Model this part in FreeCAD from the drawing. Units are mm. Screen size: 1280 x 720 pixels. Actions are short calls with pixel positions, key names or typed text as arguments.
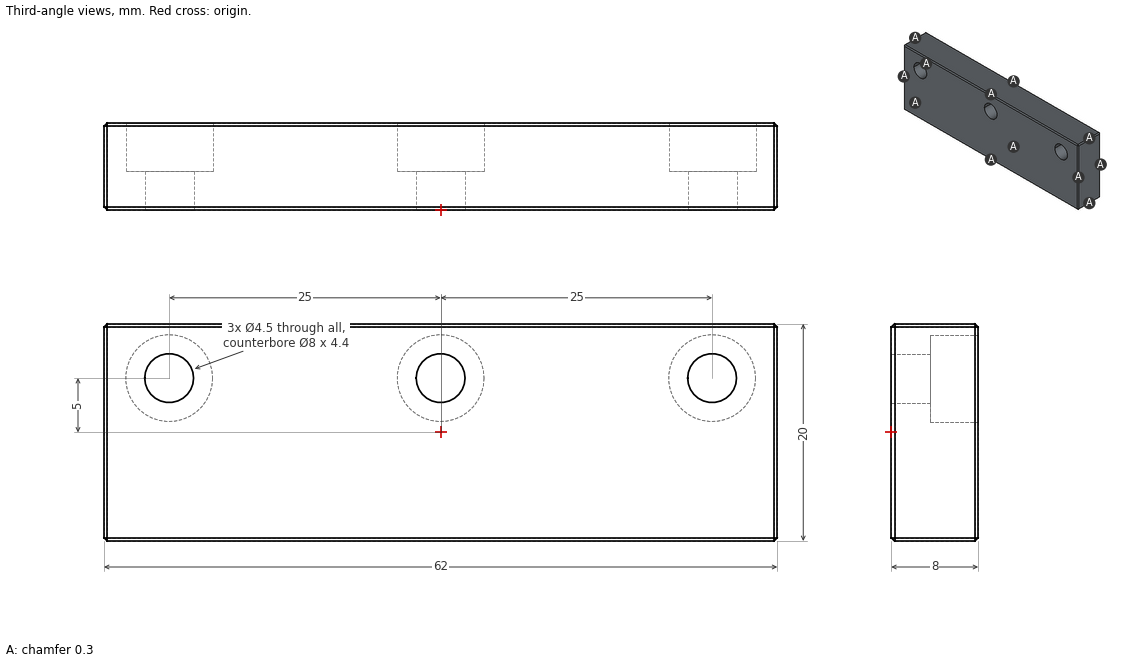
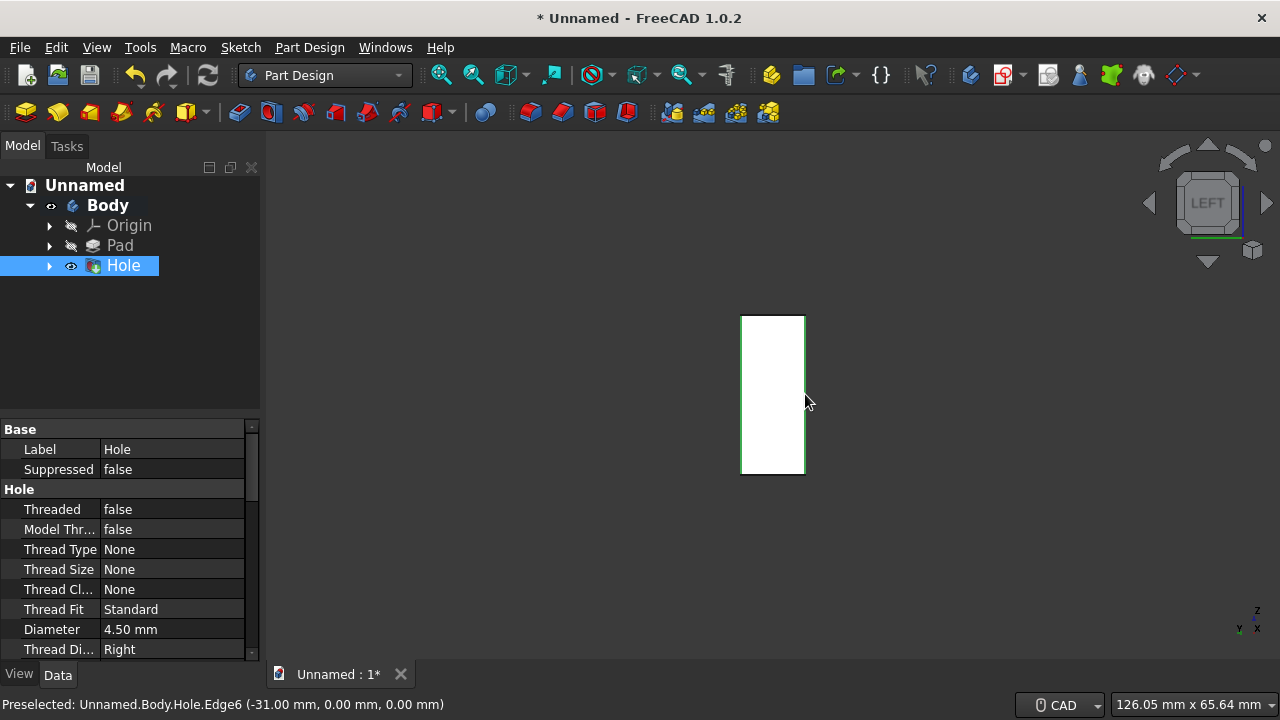
click(564, 112)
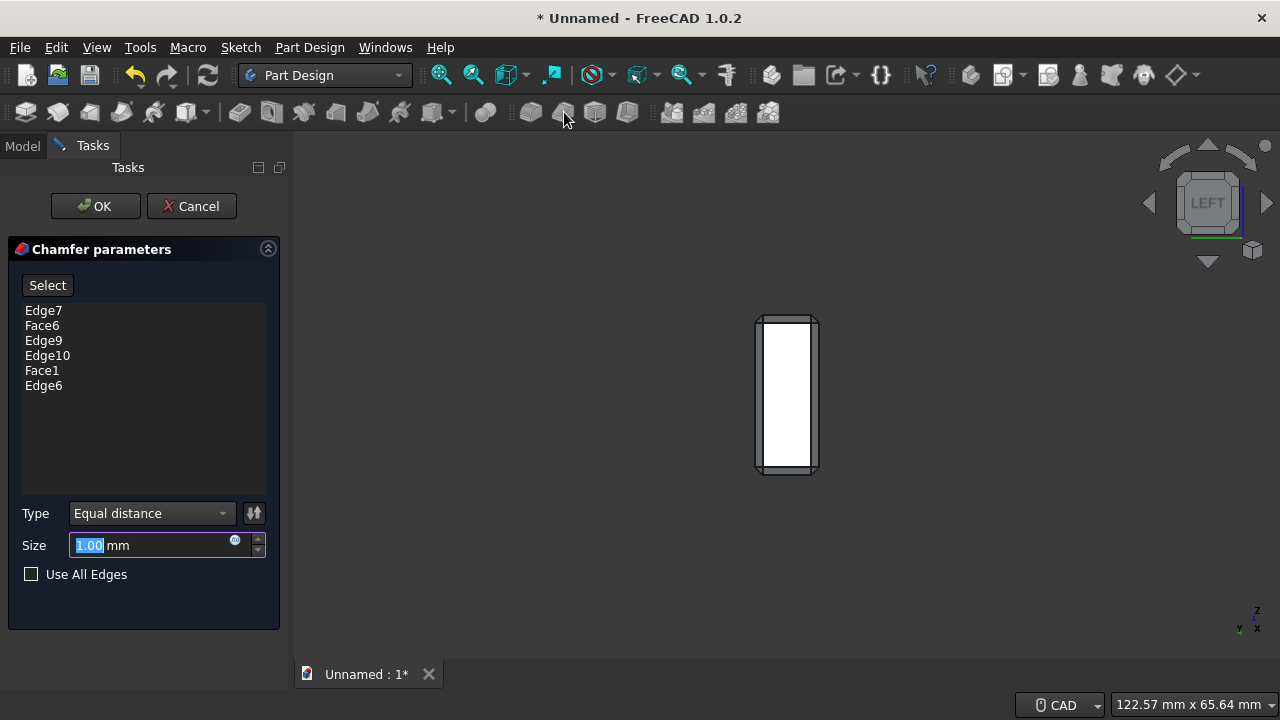
text(0.3)
key(Tab)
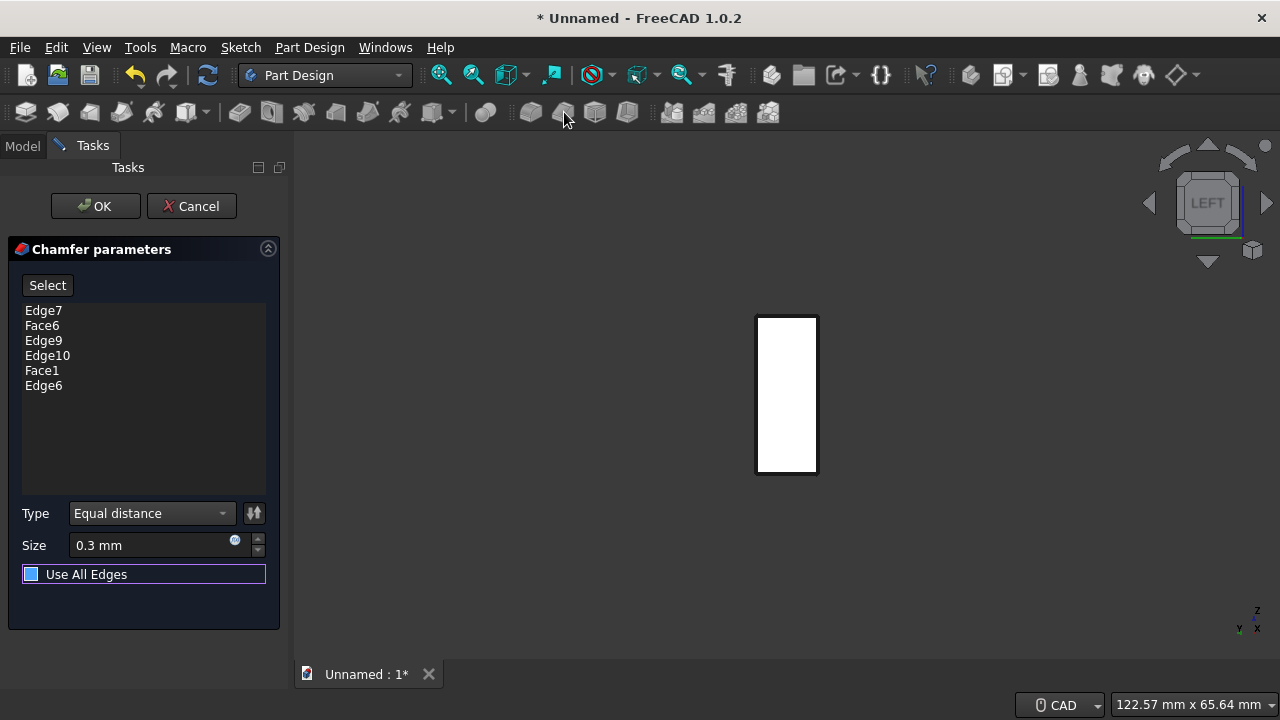
click(96, 206)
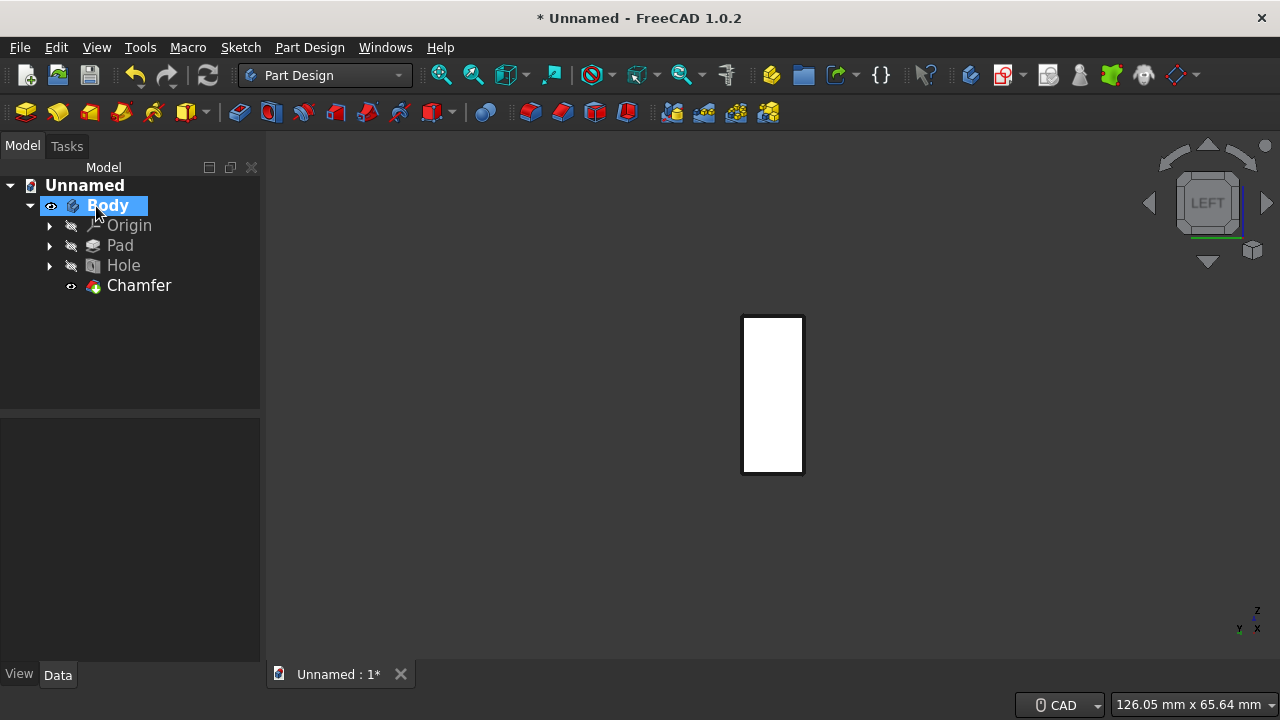
key(0)